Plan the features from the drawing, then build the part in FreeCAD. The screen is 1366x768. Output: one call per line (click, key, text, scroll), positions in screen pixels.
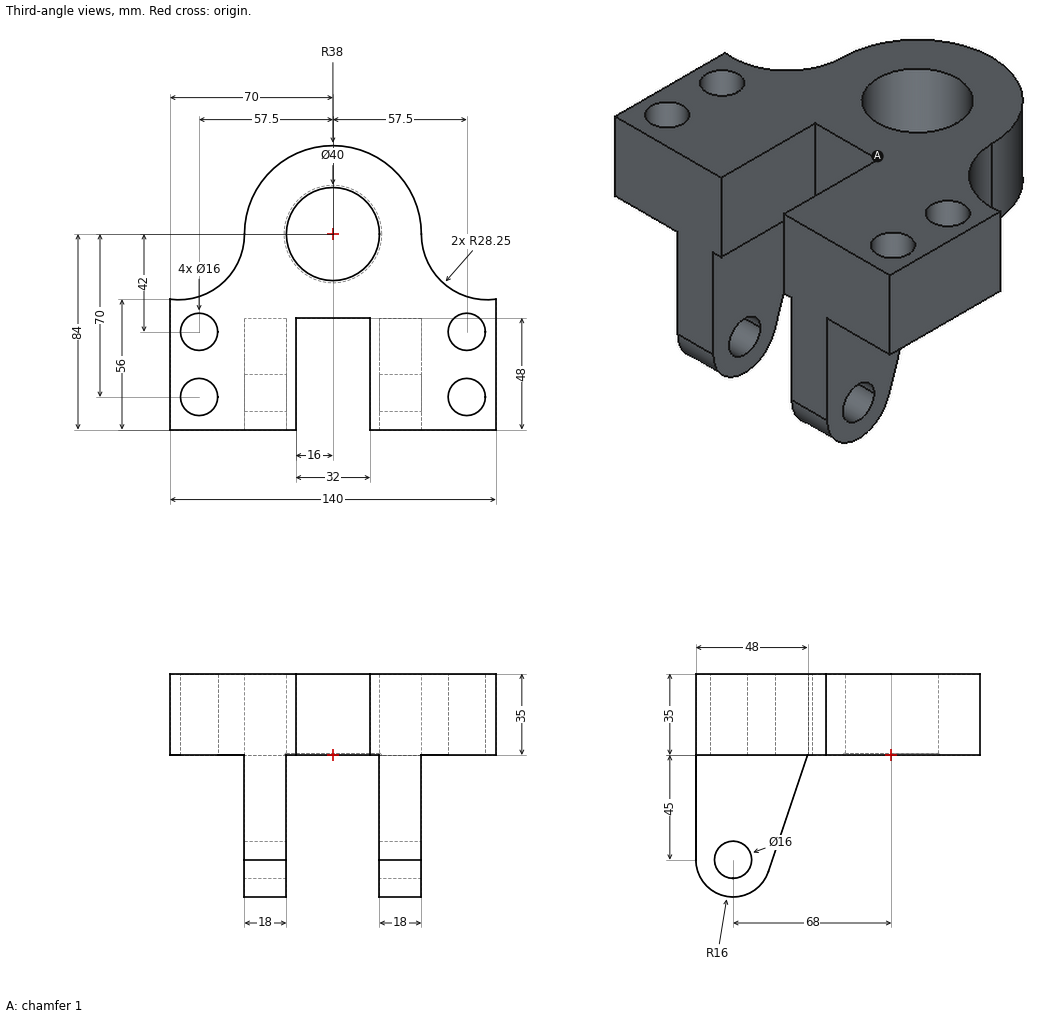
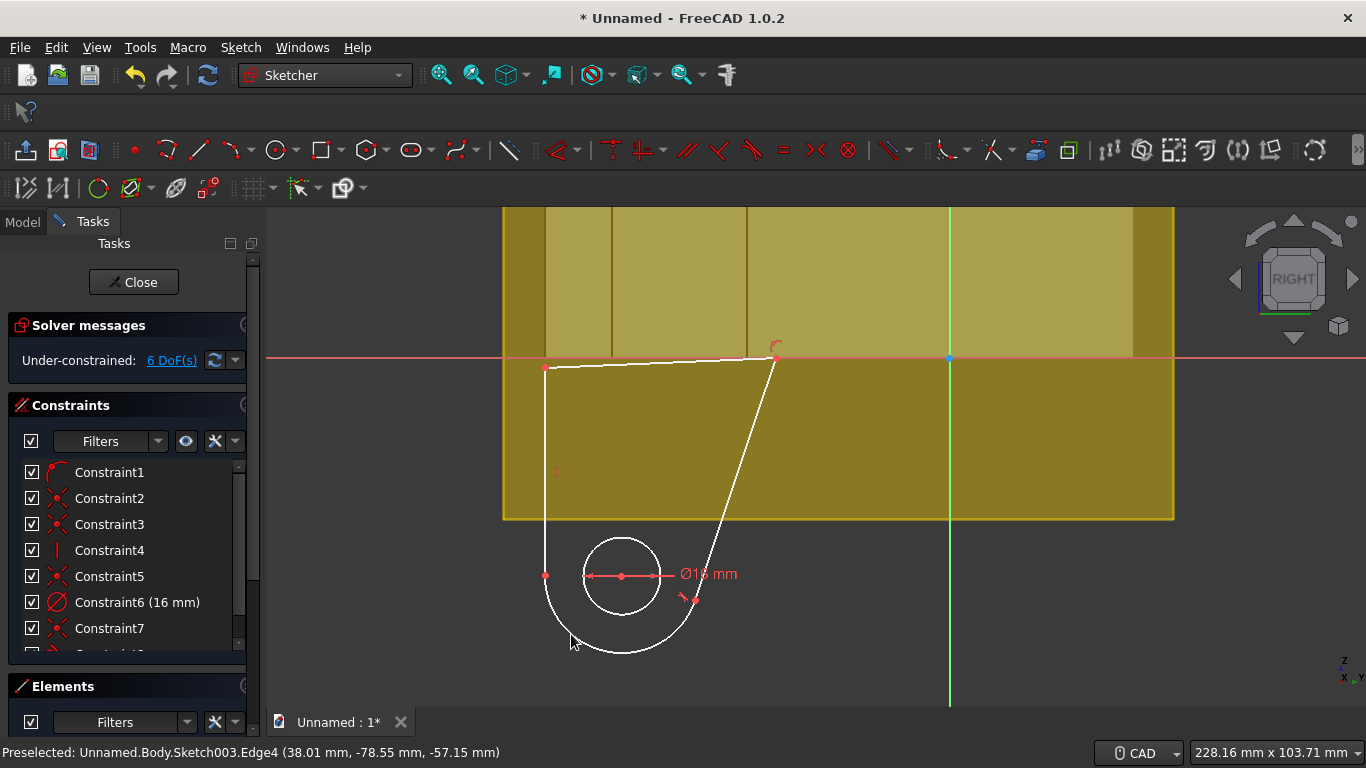
click(545, 430)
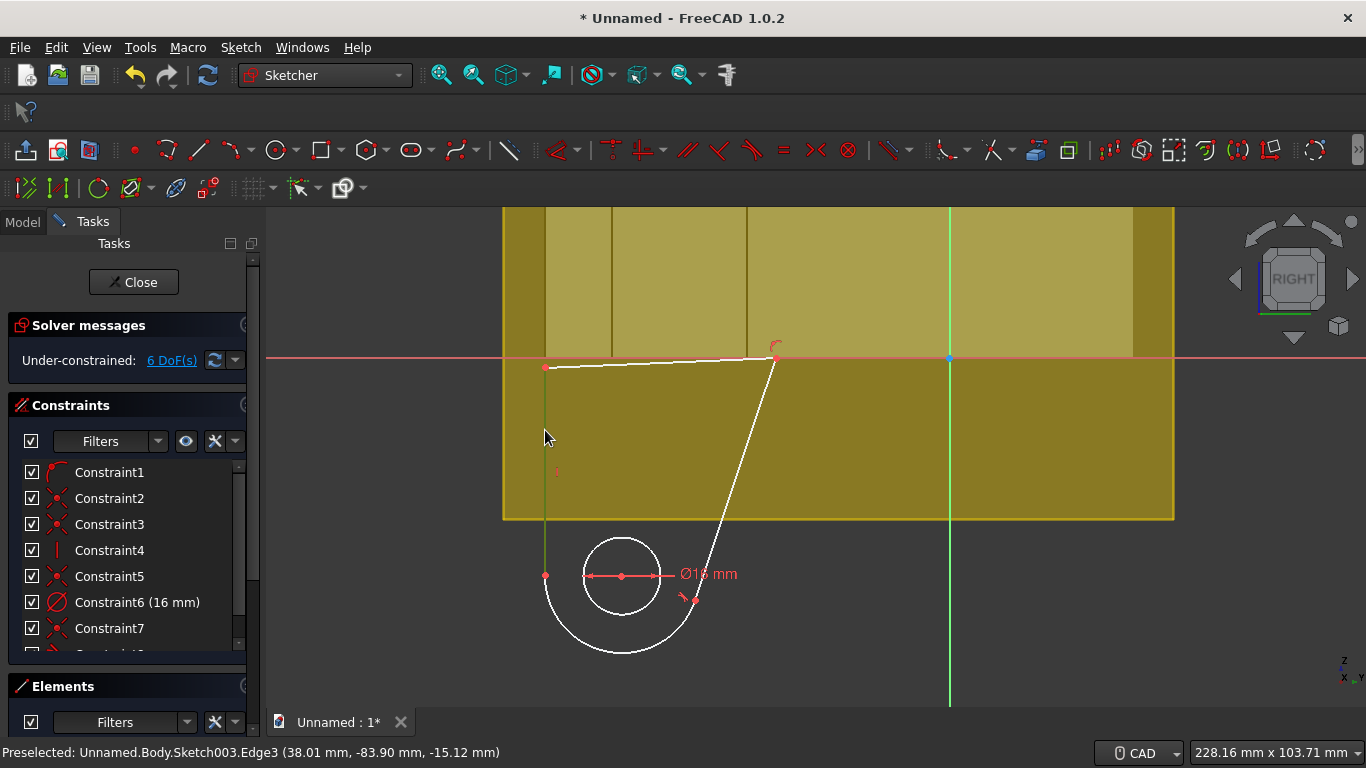
click(571, 634)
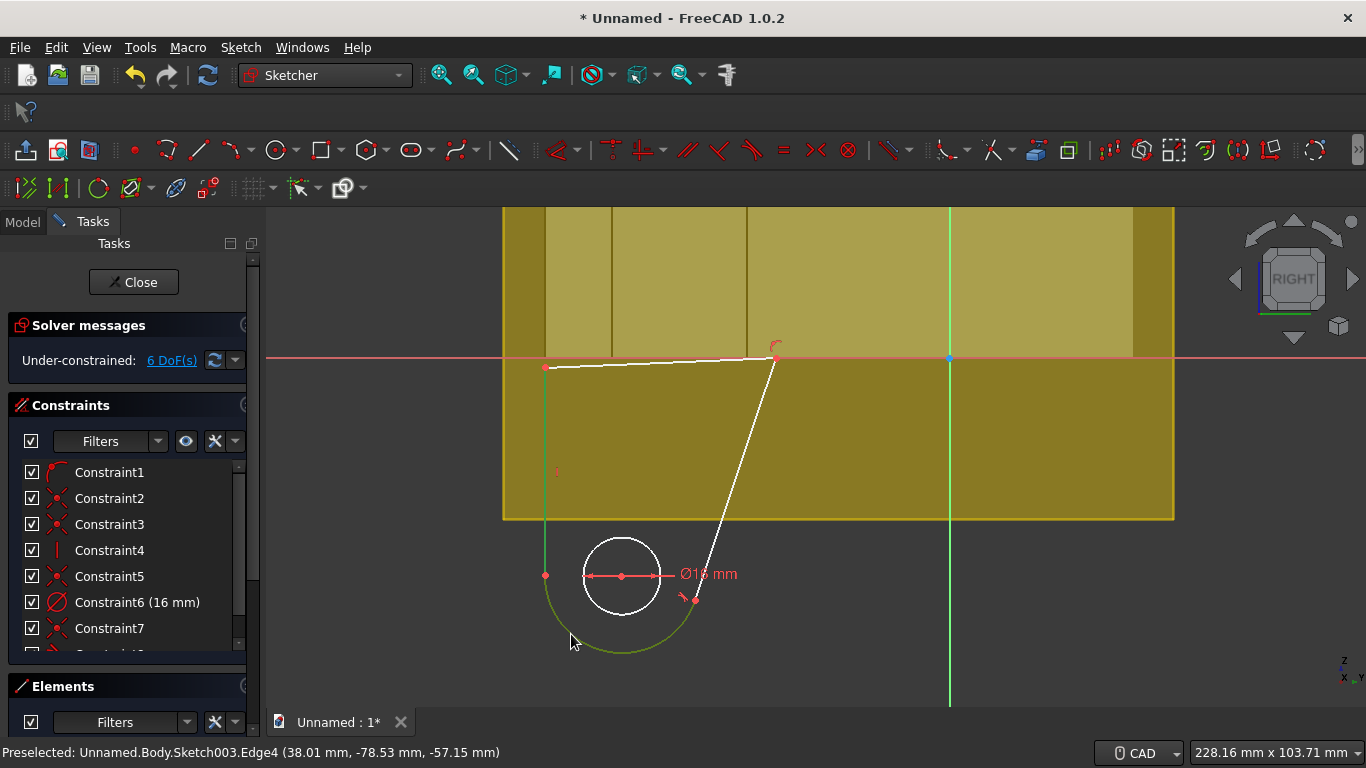
key(t)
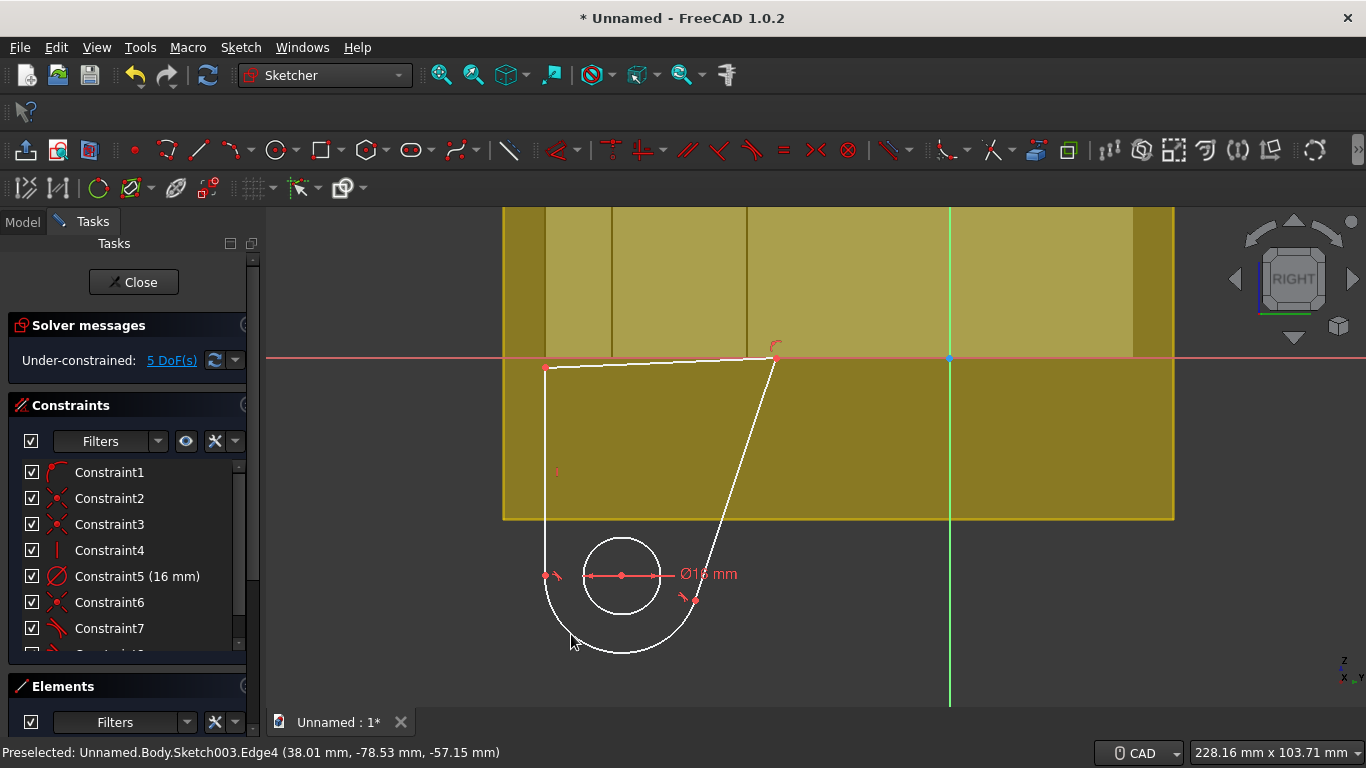
click(707, 361)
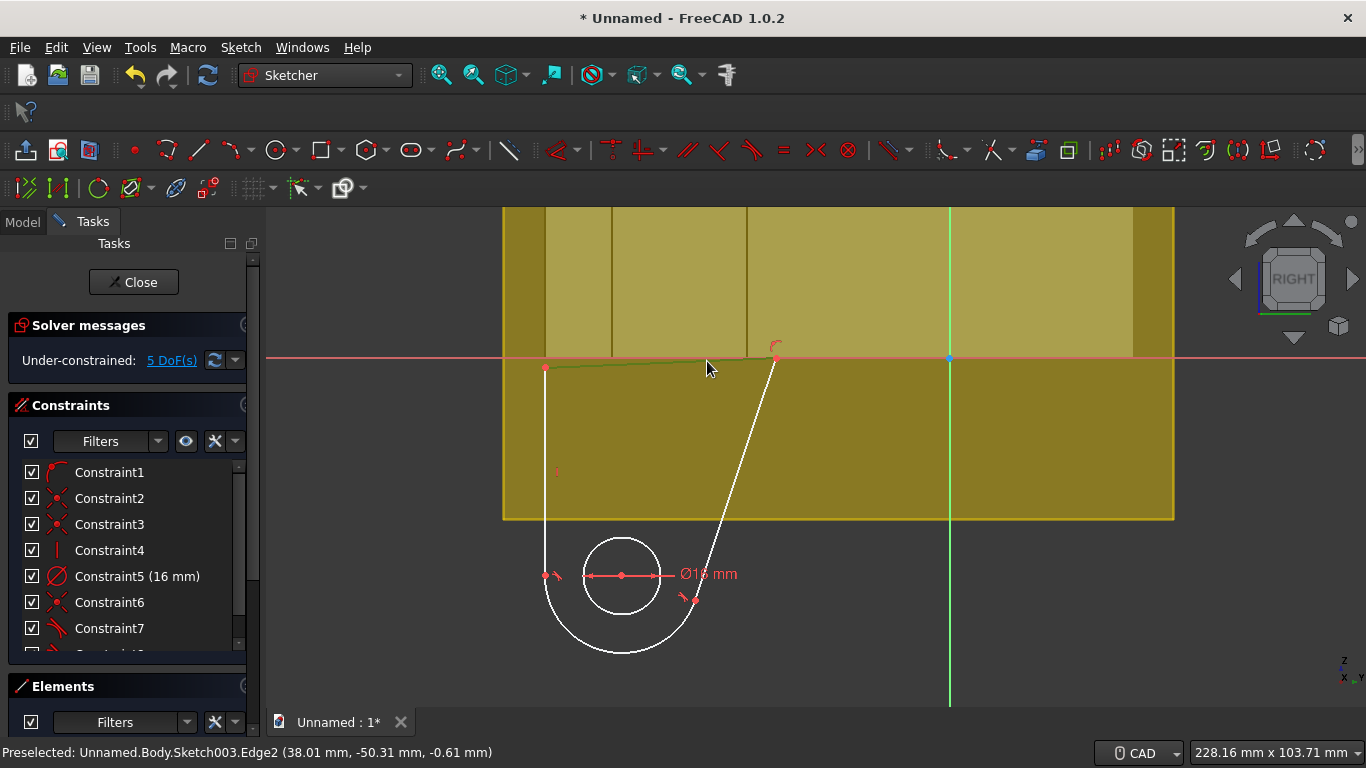
click(666, 150)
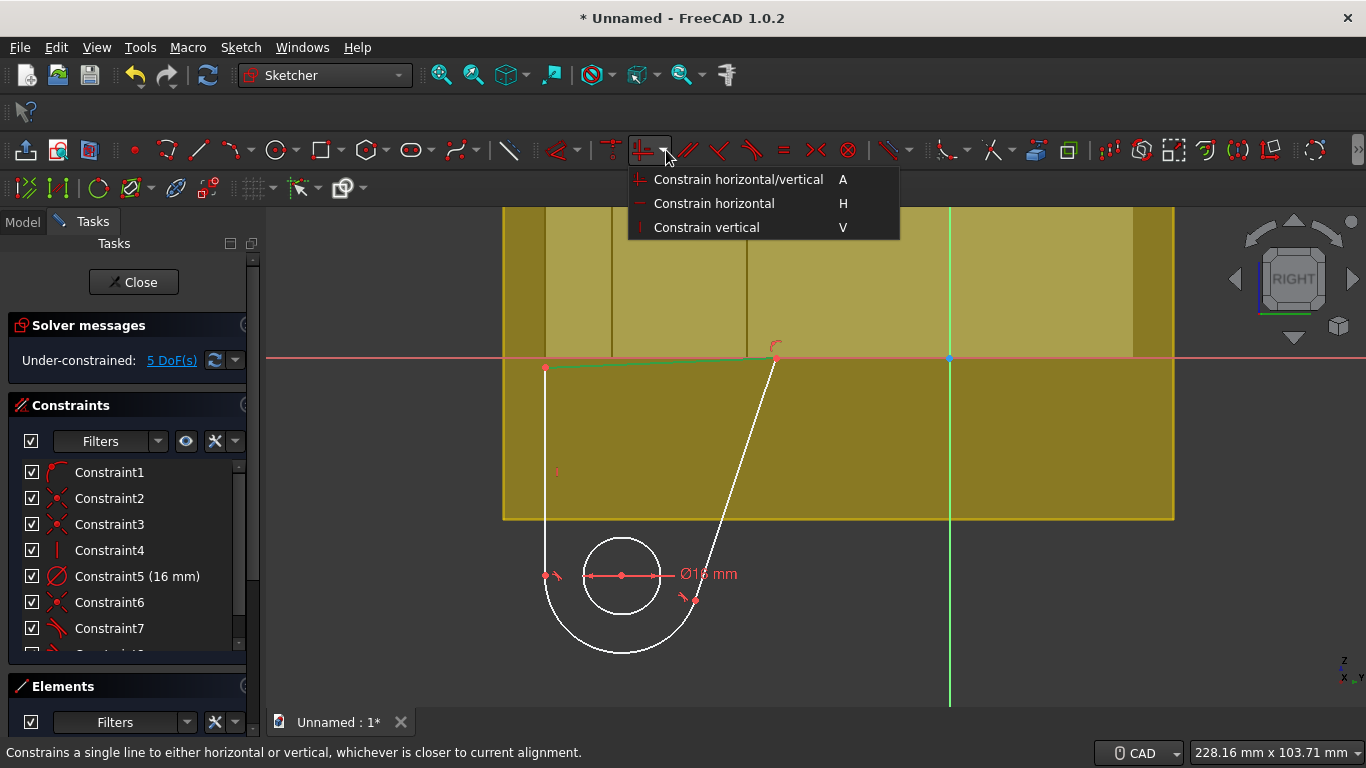
click(764, 203)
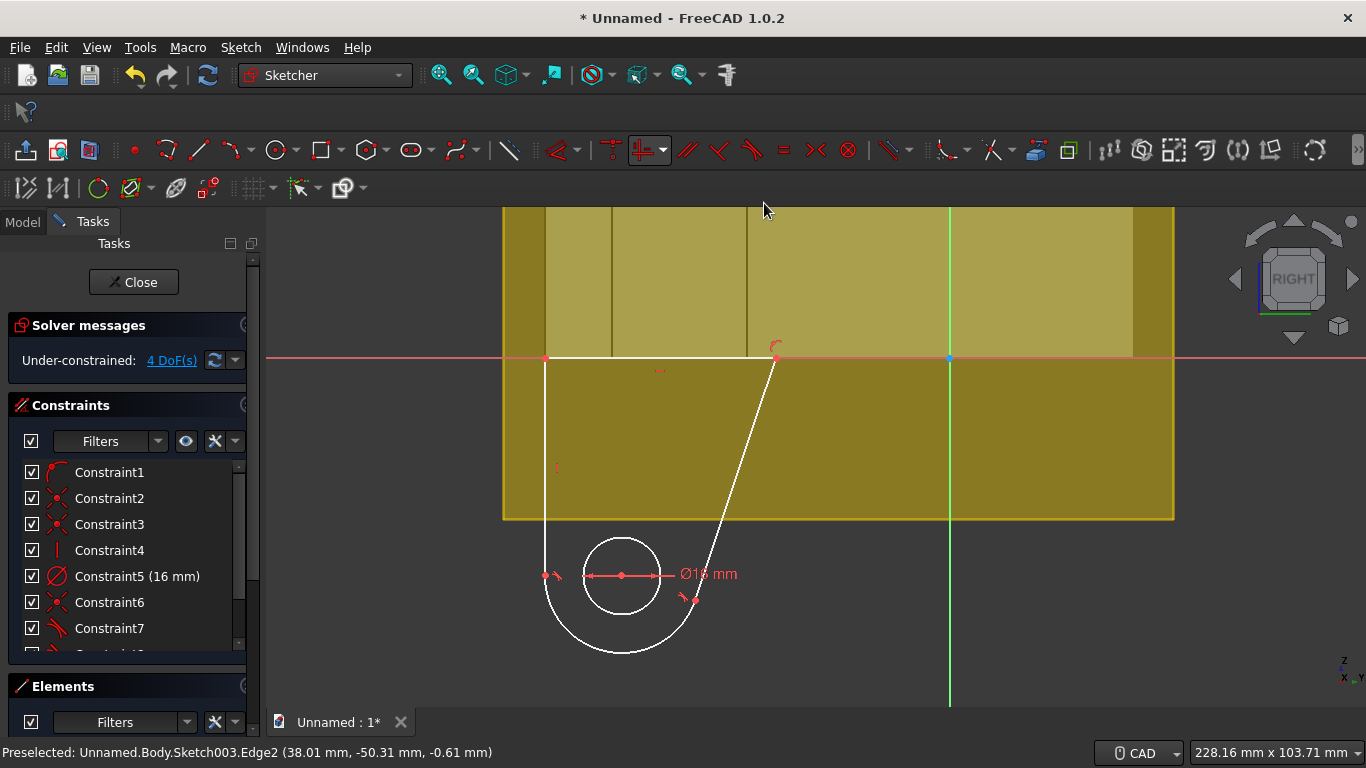
key(d)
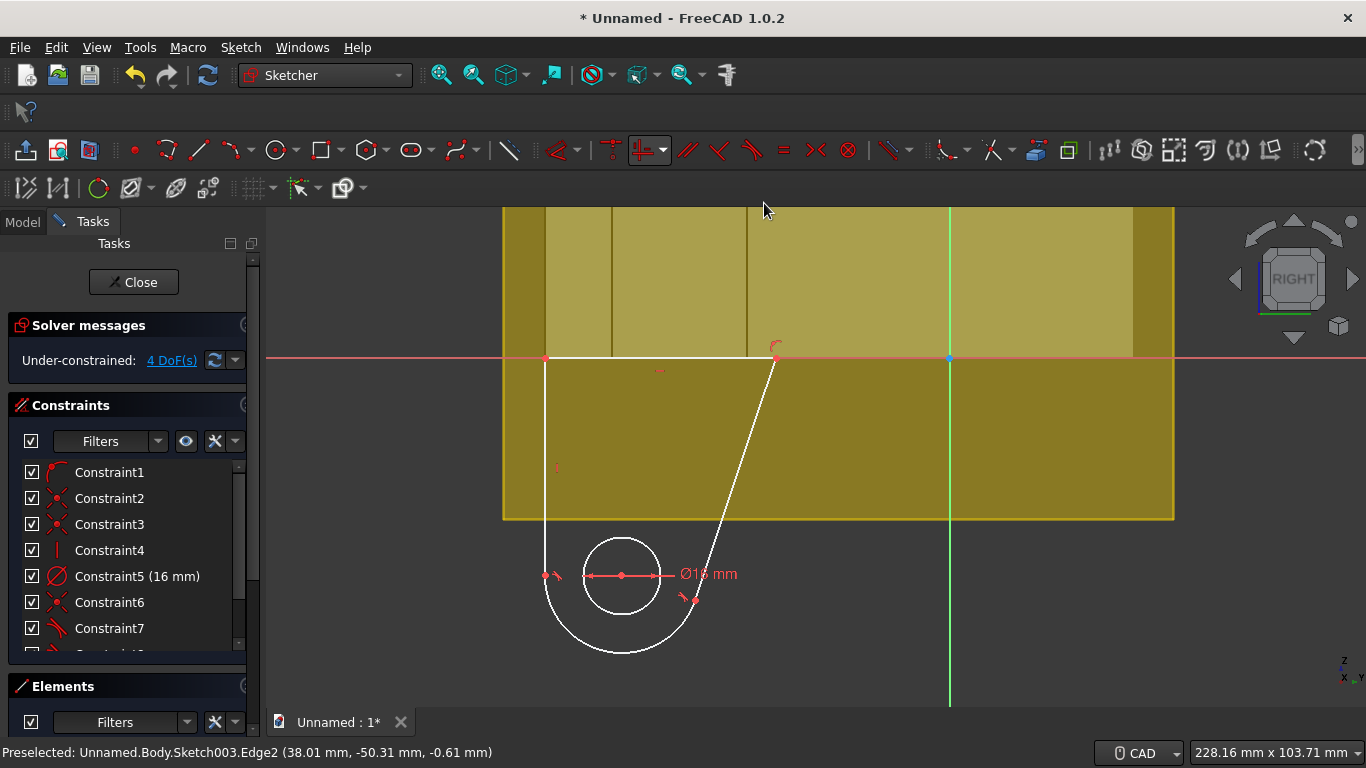
click(571, 634)
click(550, 658)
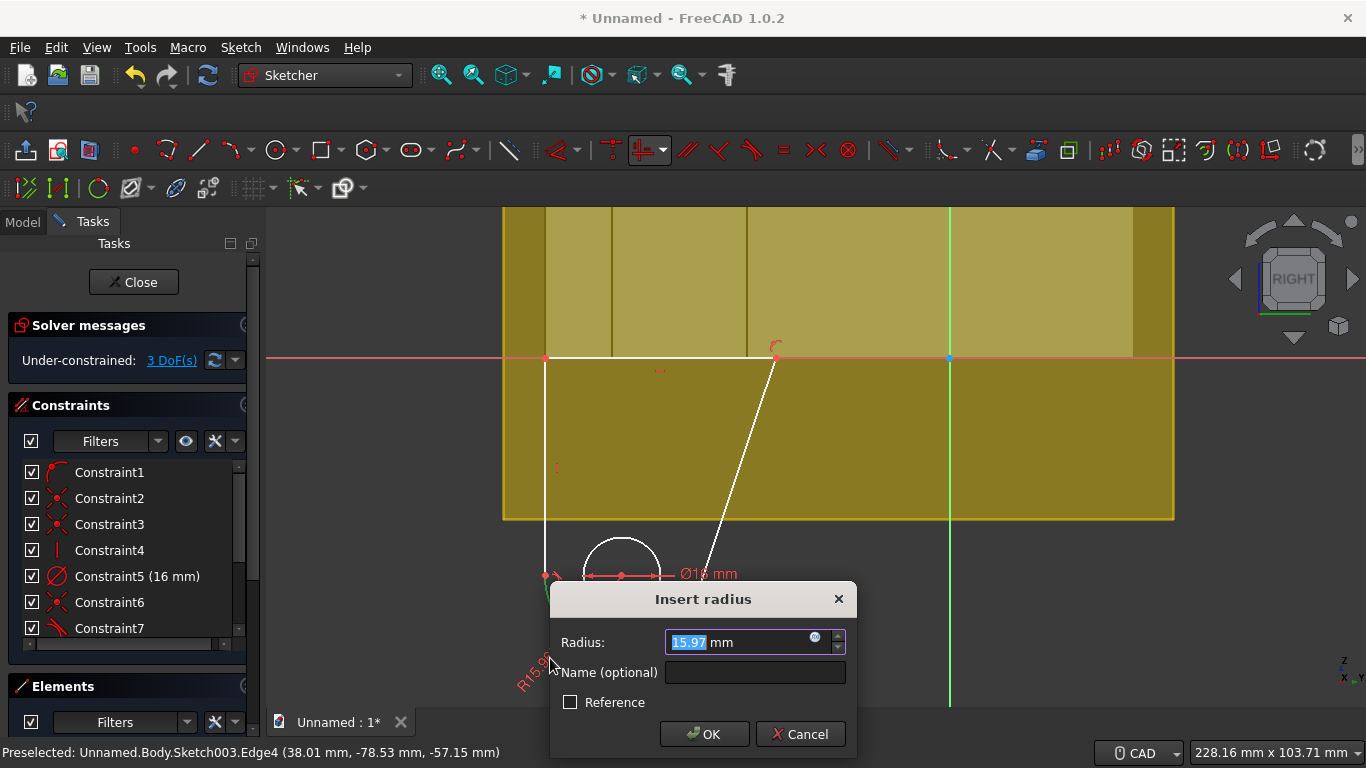
text(16)
key(Return)